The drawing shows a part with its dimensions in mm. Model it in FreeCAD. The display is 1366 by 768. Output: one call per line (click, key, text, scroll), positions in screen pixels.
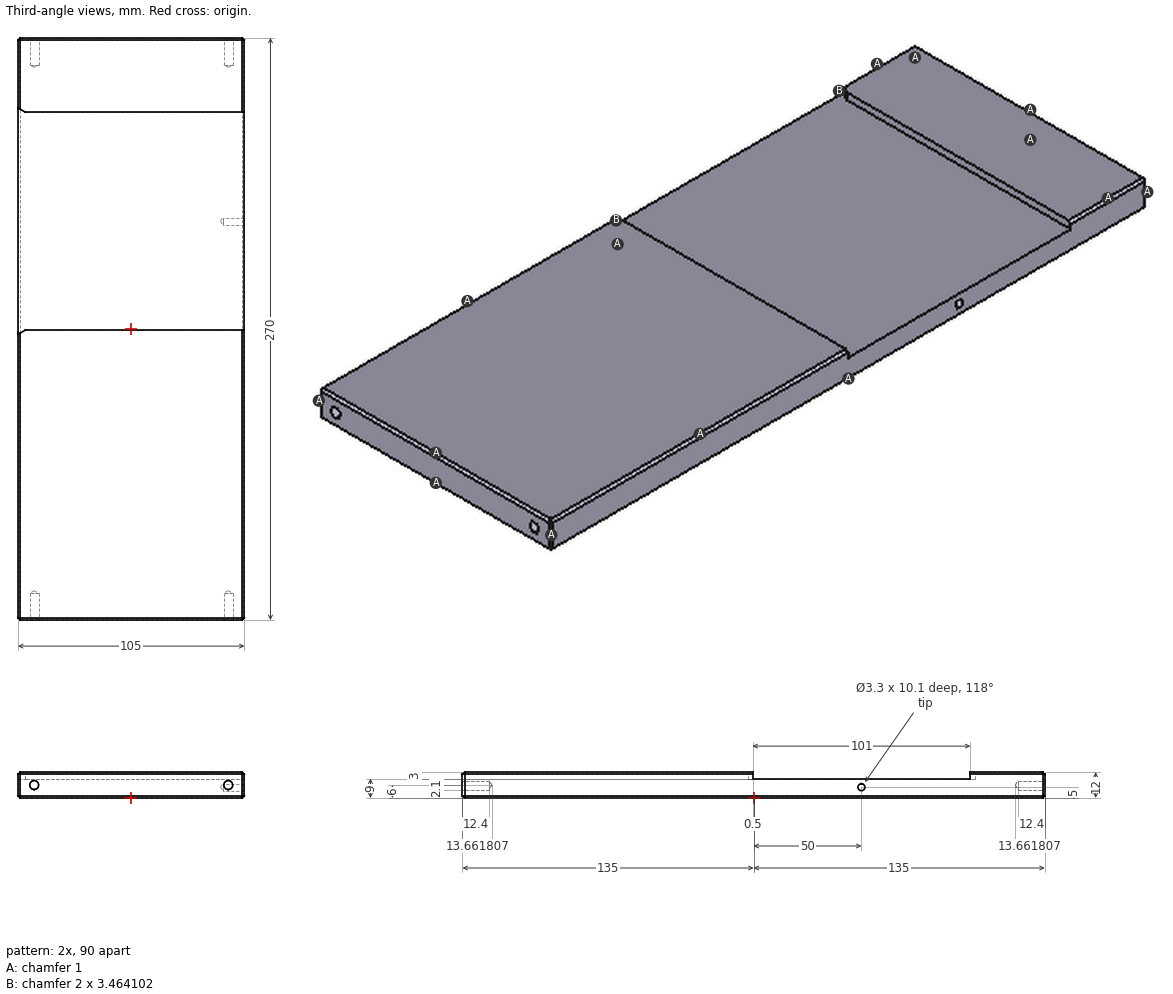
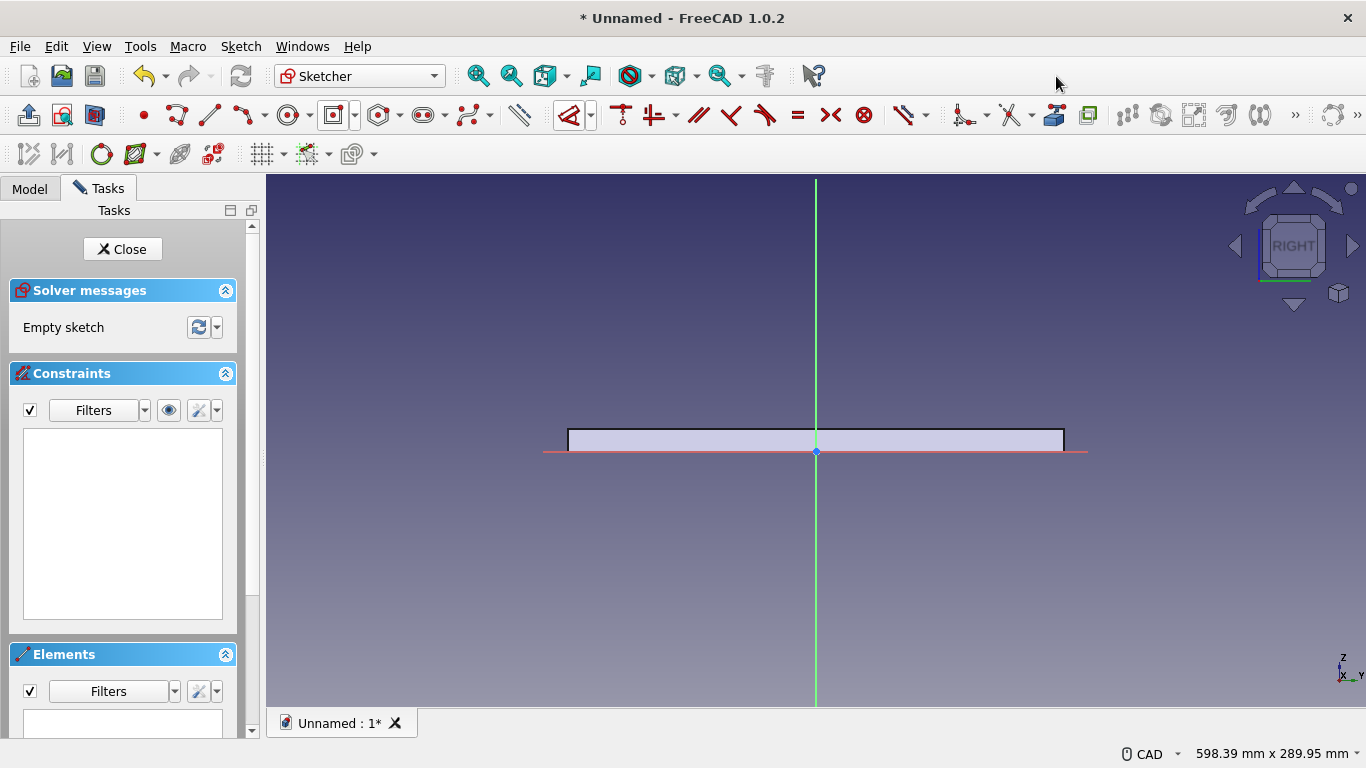
scroll(977, 440, up, 6)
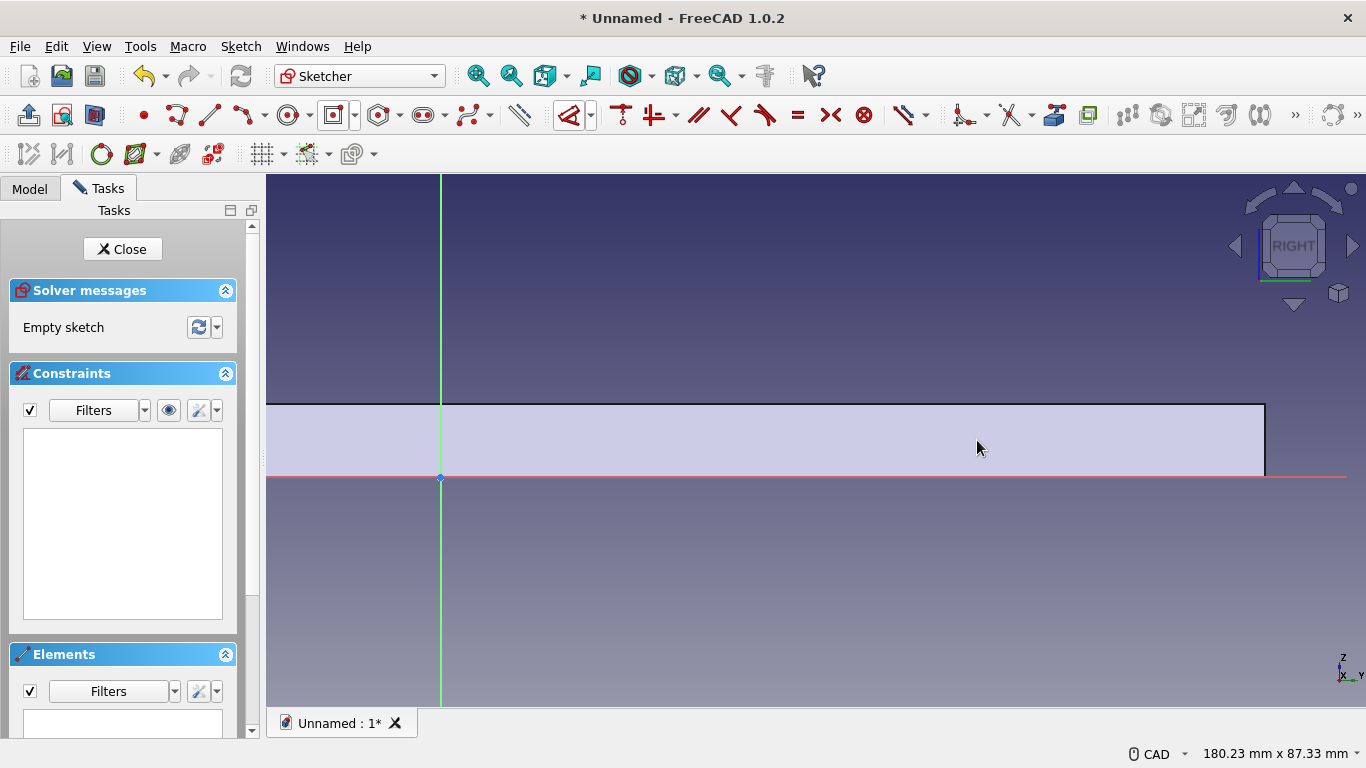
key(g)
key(r)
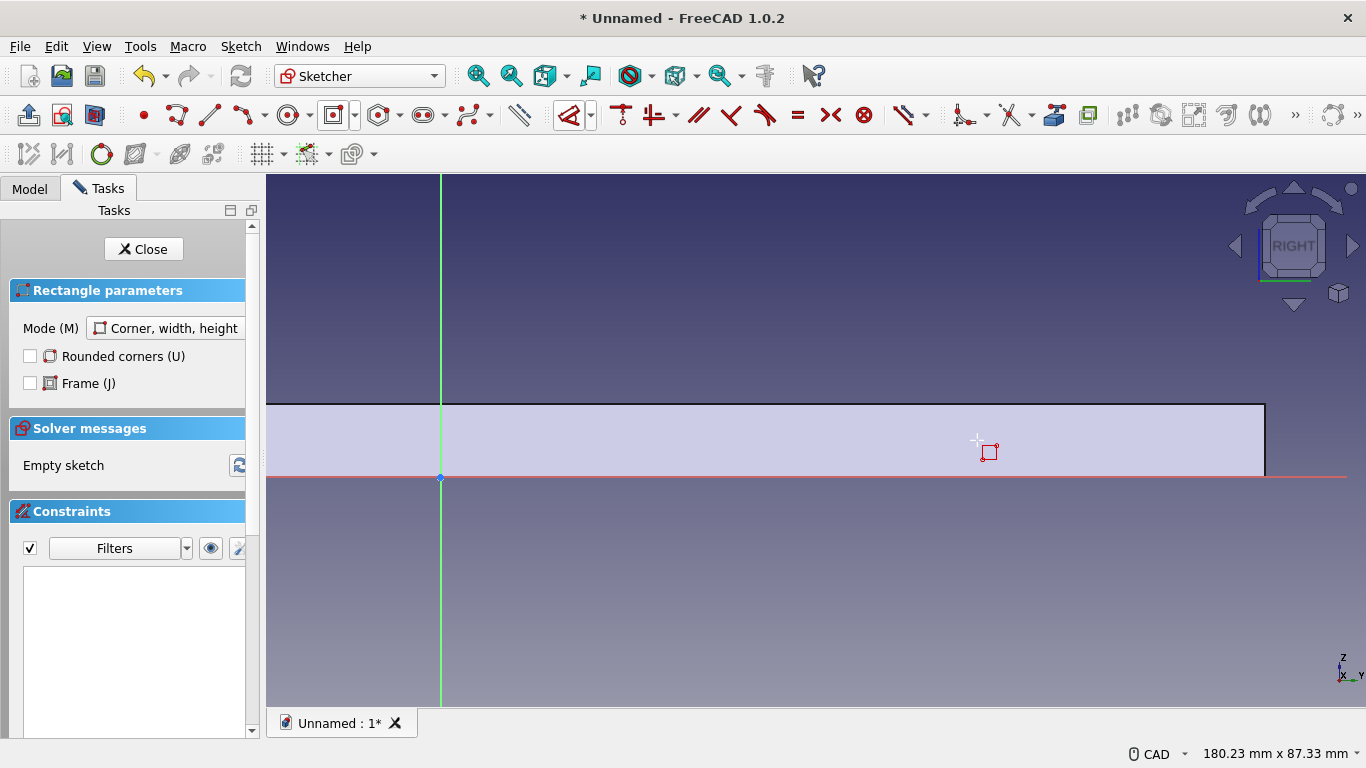
scroll(438, 404, up, 9)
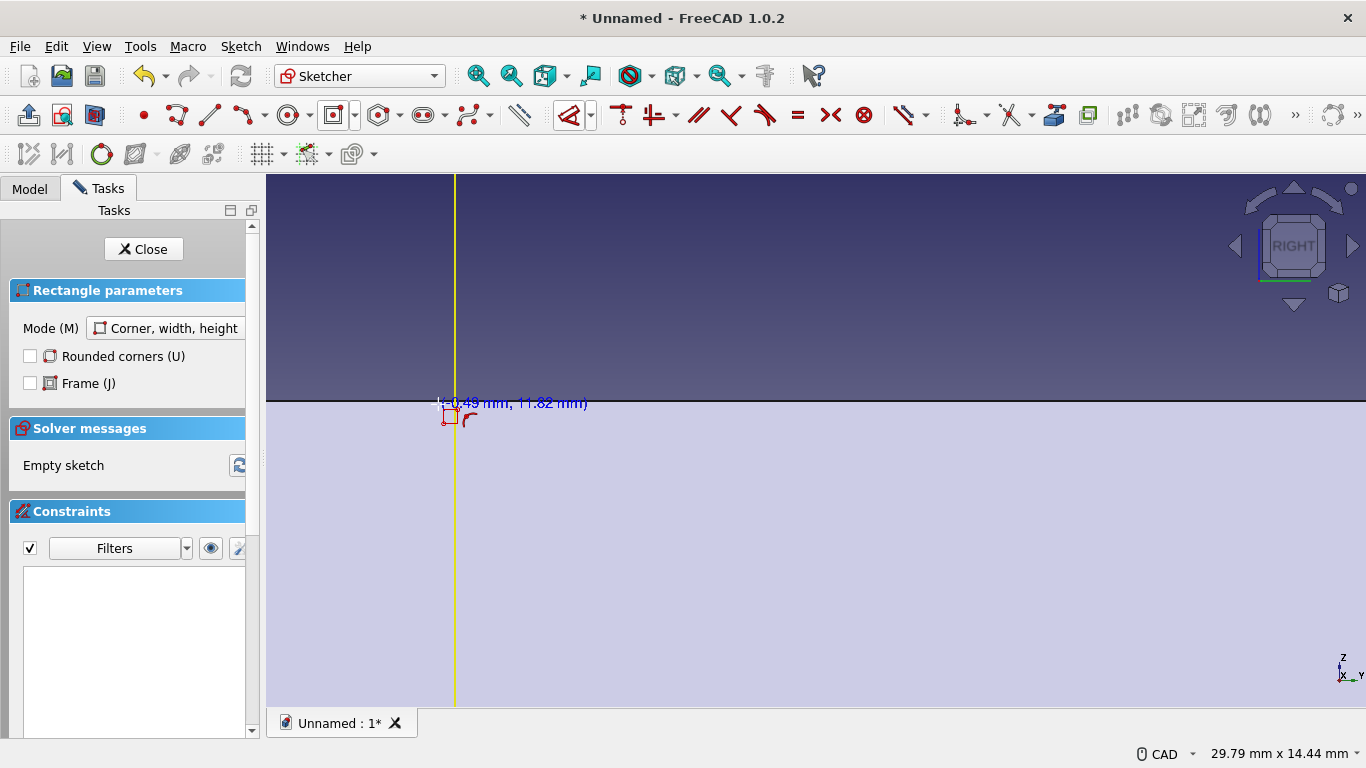
click(437, 401)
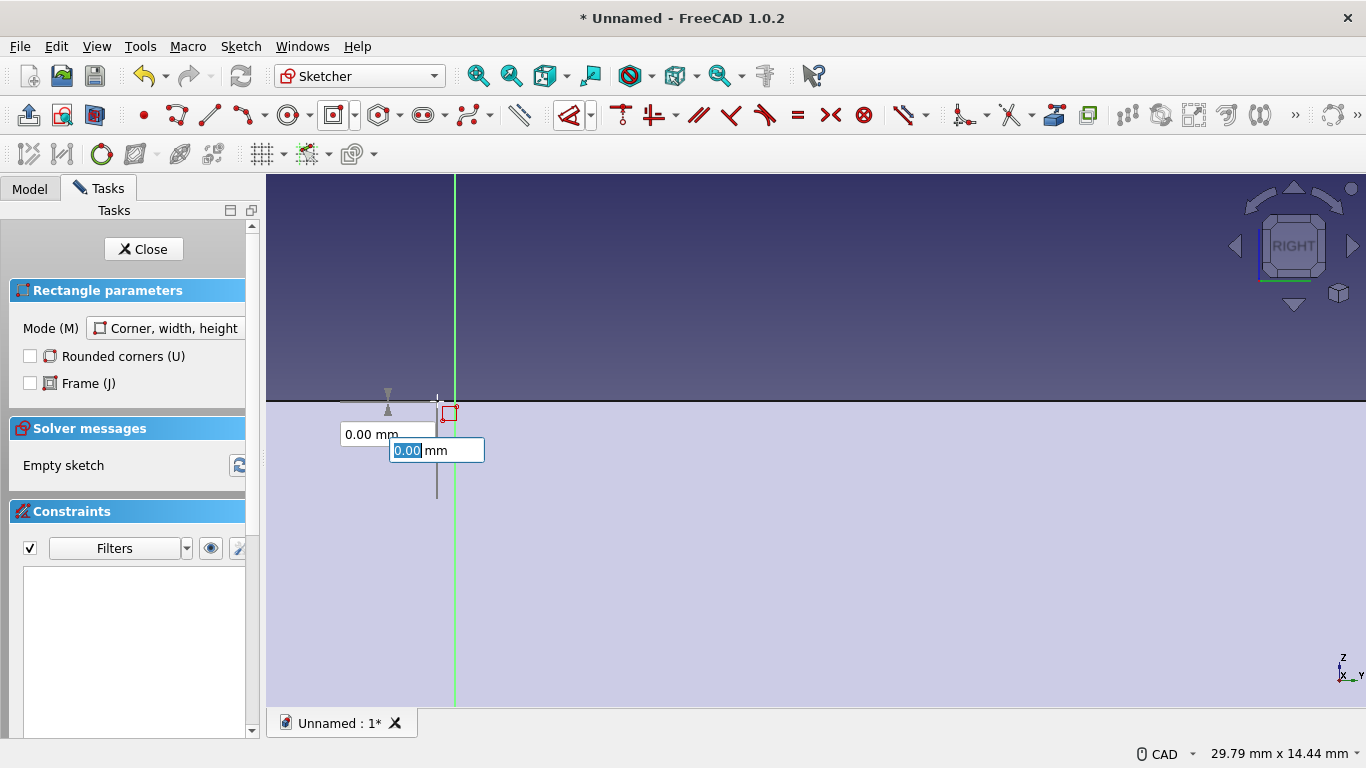
scroll(440, 404, down, 9)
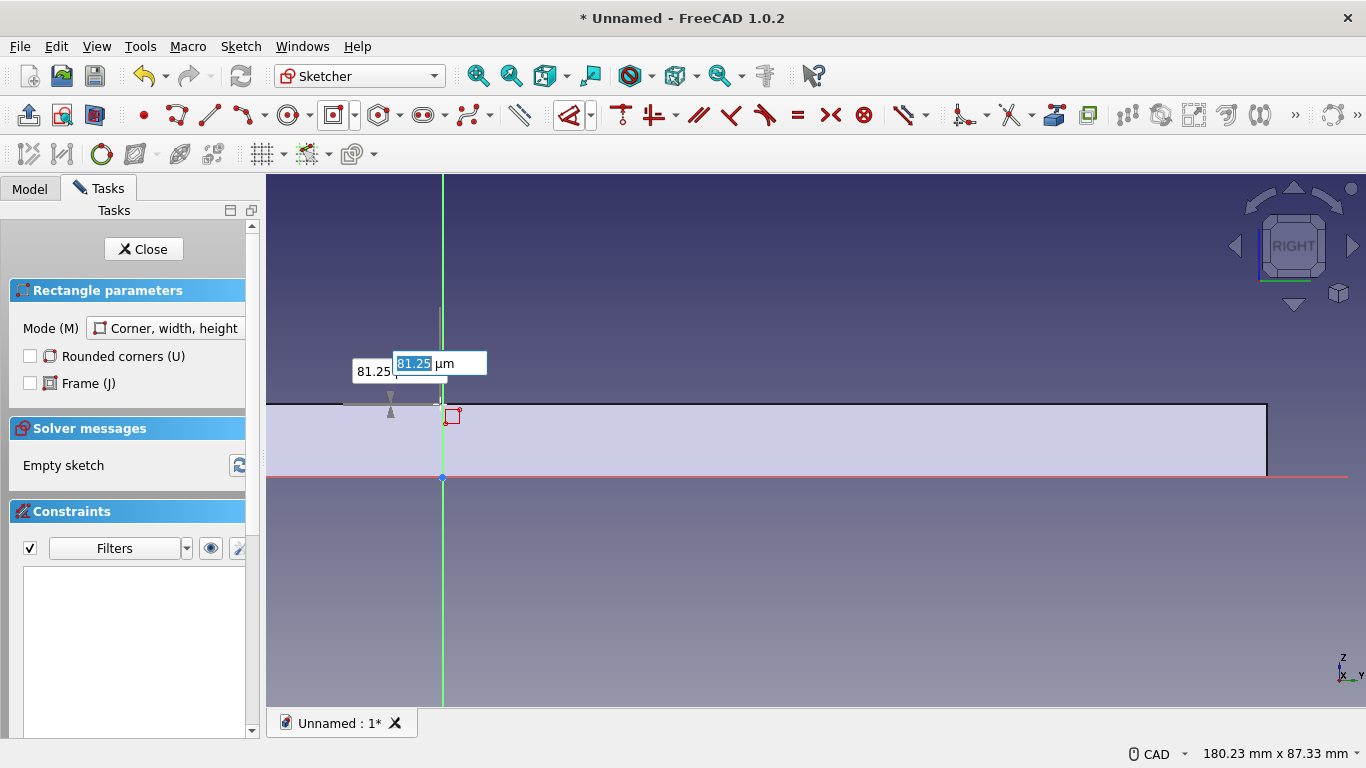
click(1056, 422)
key(Escape)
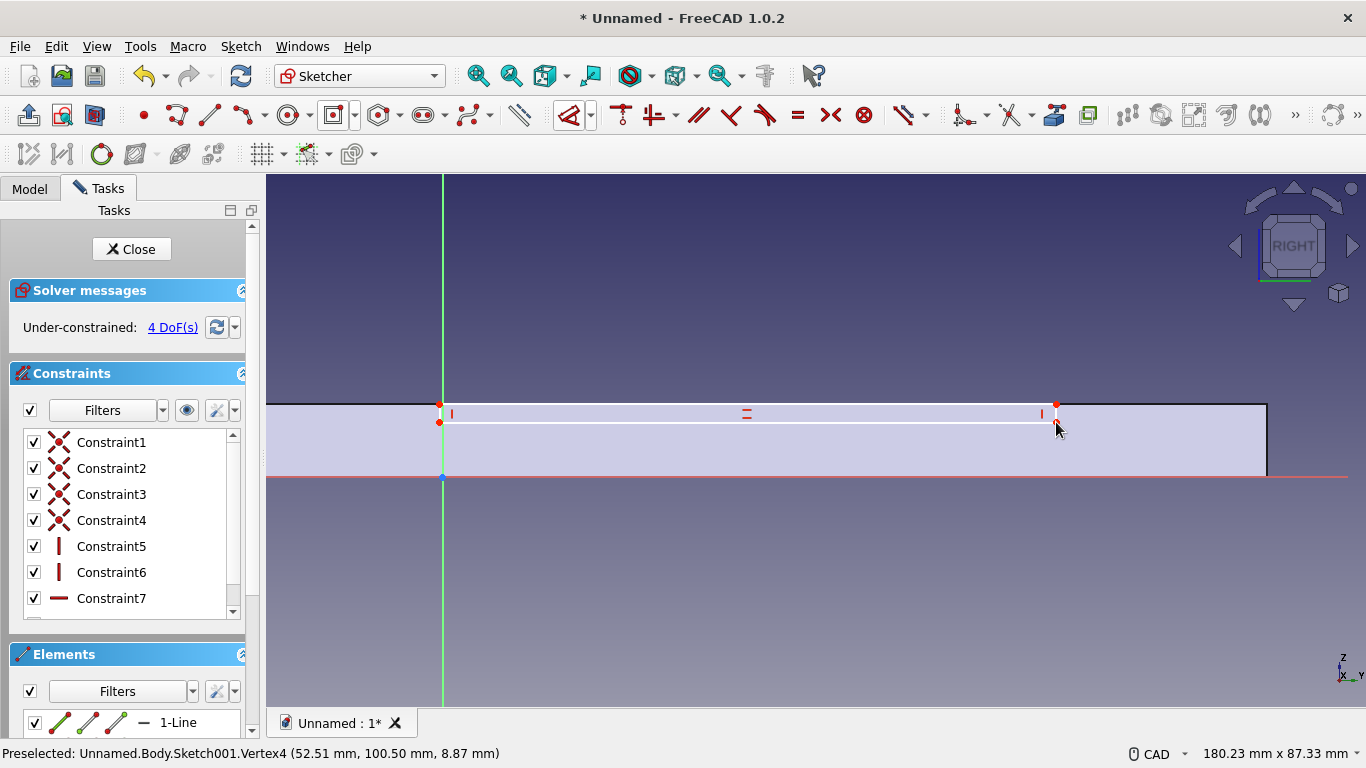
click(568, 116)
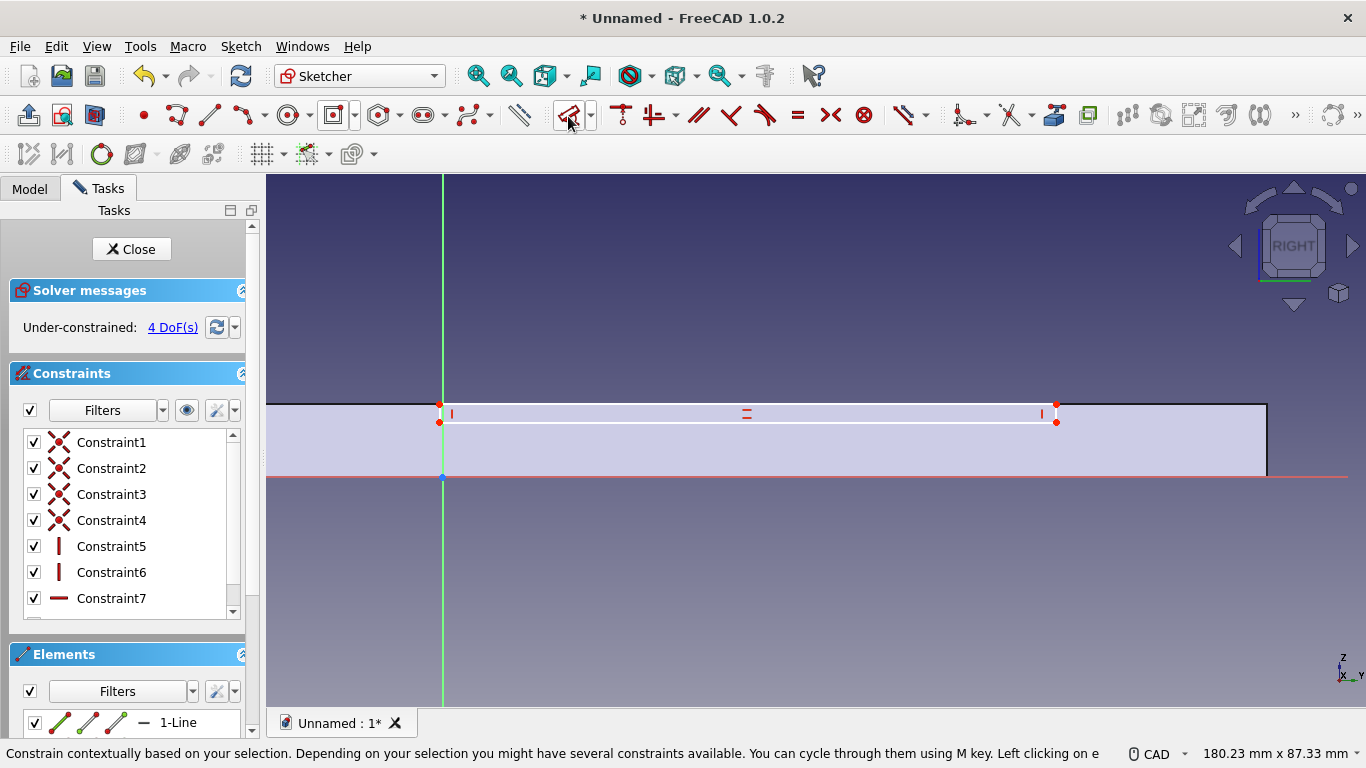
scroll(440, 414, up, 4)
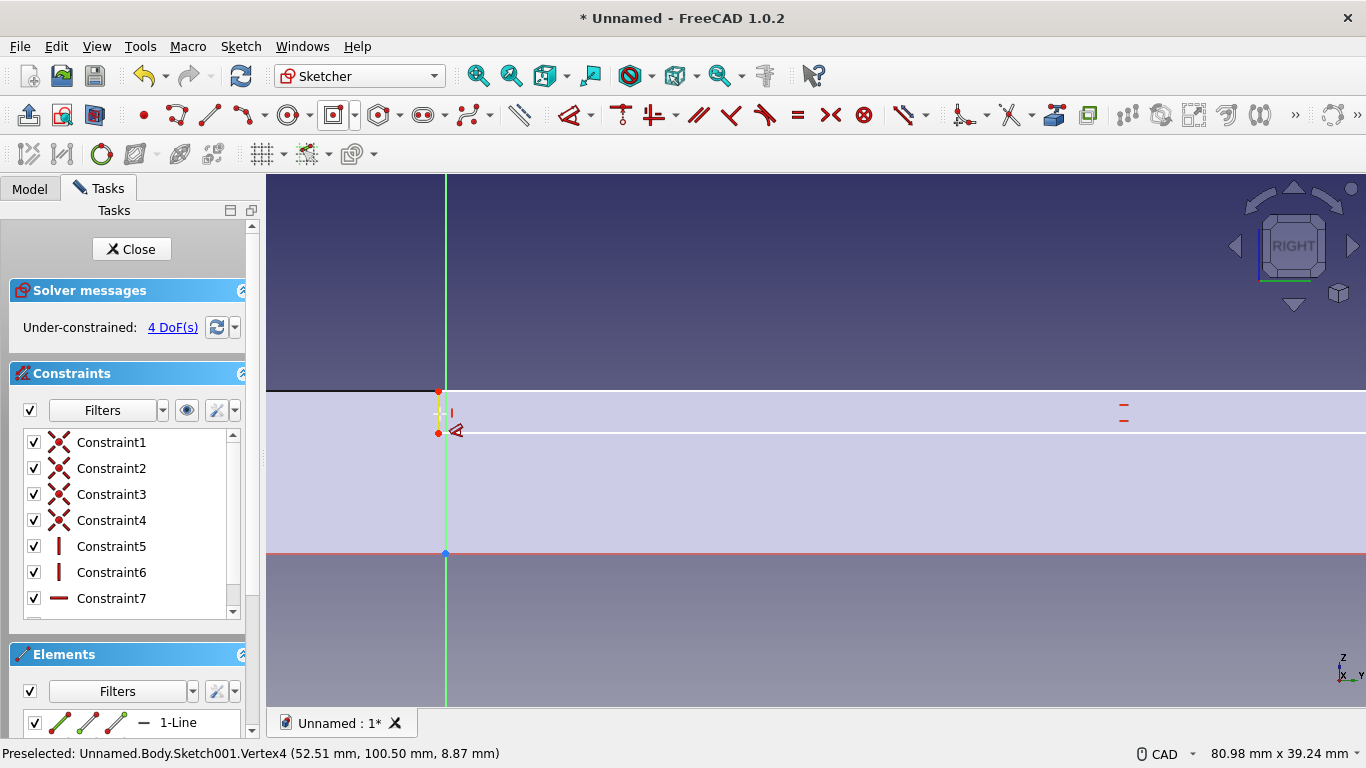
click(439, 412)
click(405, 412)